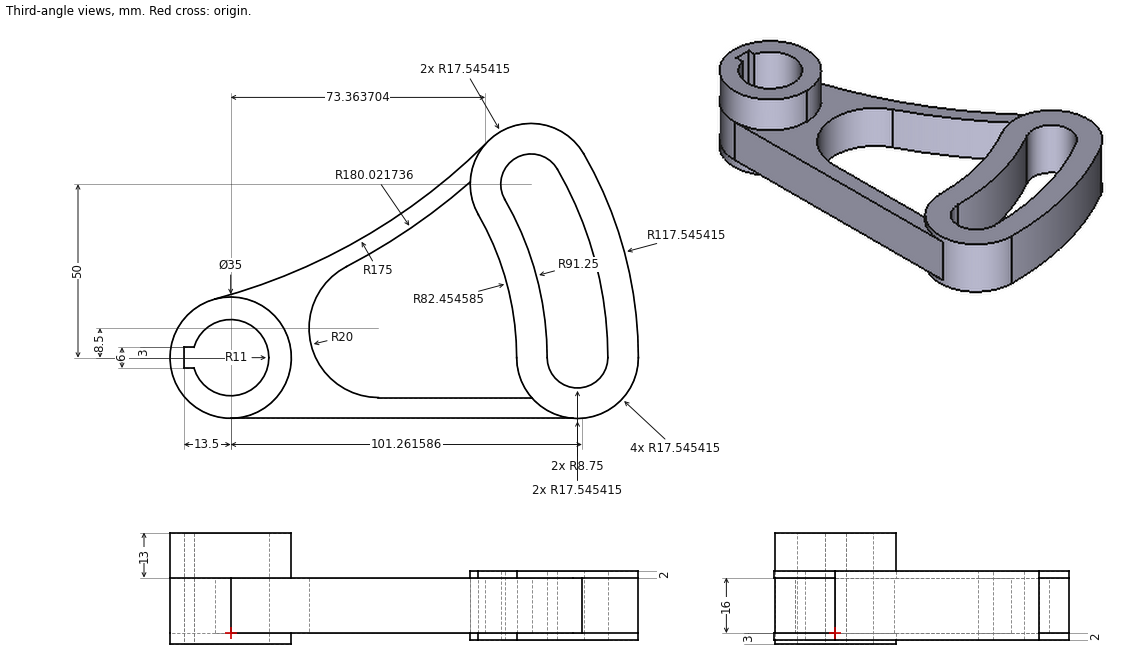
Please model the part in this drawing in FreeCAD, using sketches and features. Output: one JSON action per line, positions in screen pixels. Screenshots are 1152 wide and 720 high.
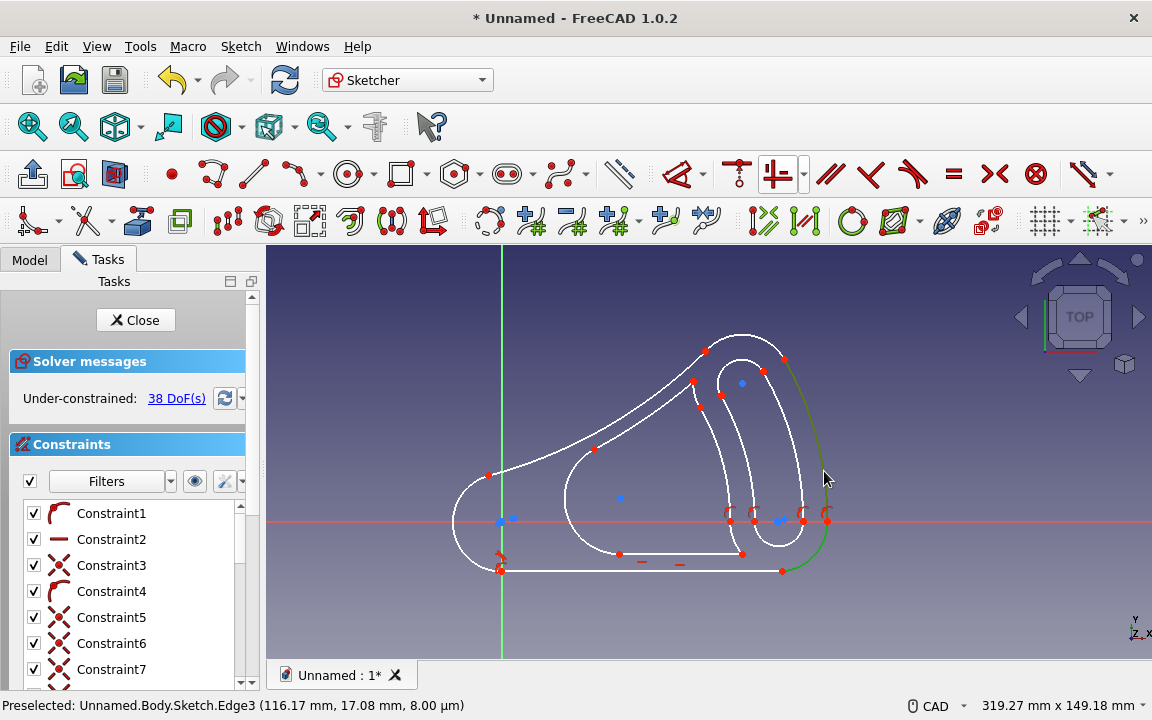
{"action": "left_click", "coordinate": [913, 174]}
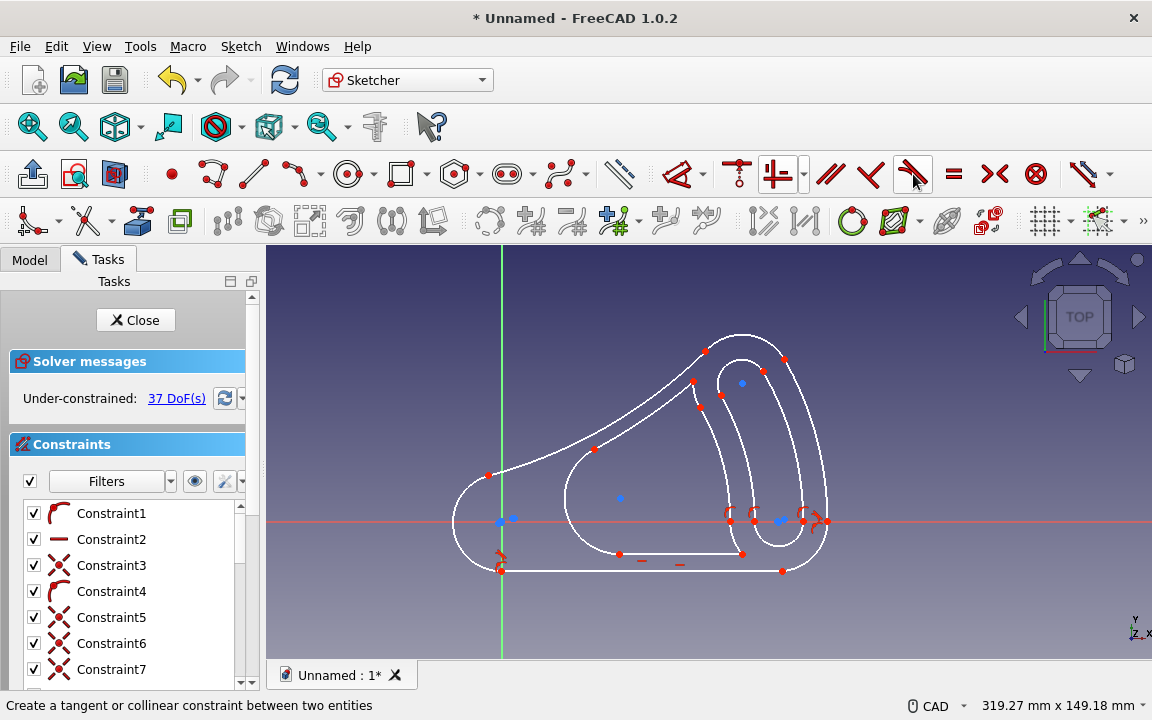
{"action": "left_click", "coordinate": [824, 471]}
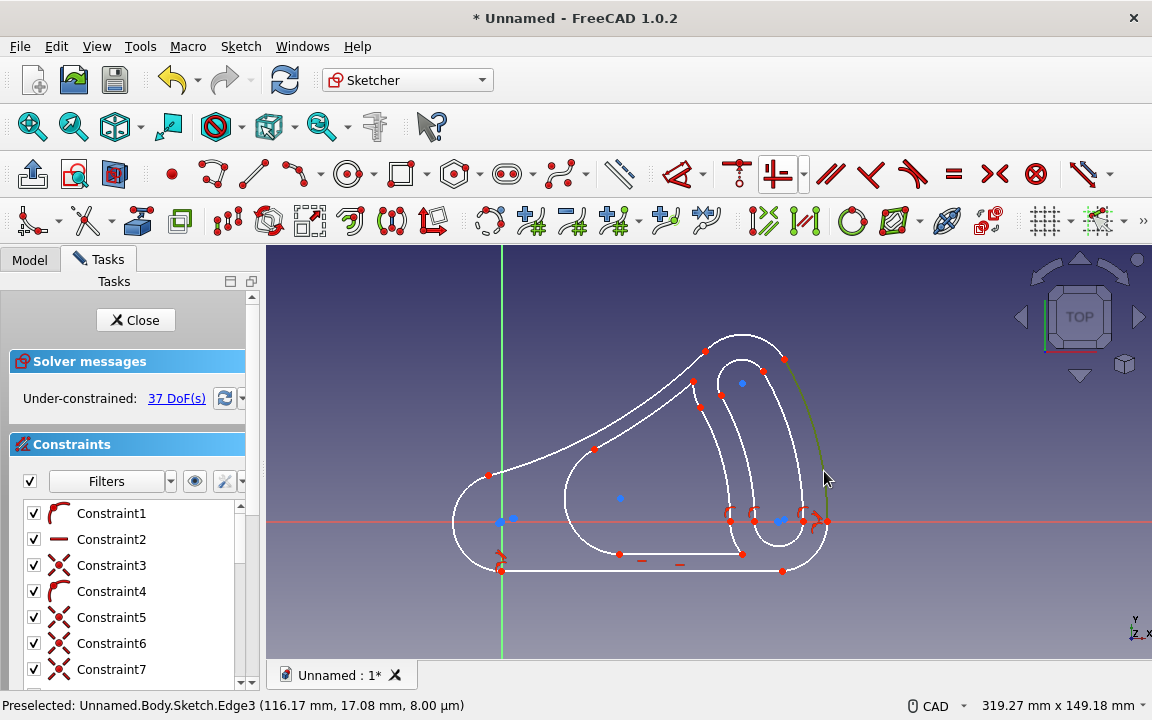
{"action": "left_click", "coordinate": [765, 340]}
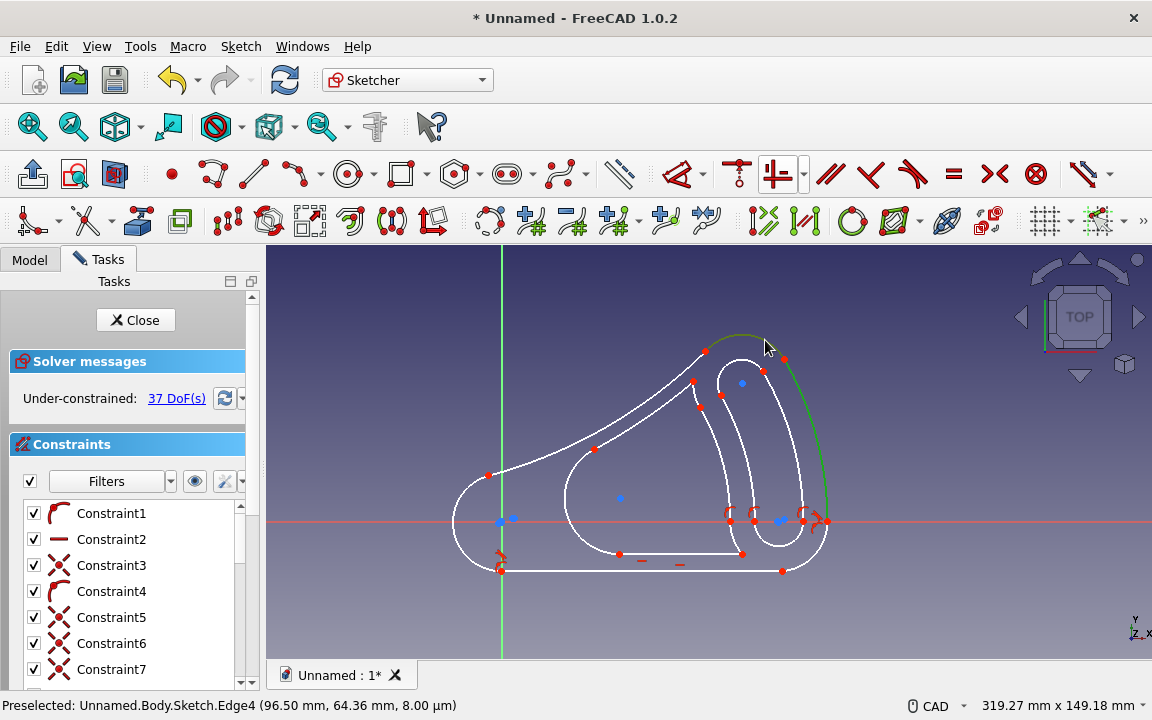
{"action": "left_click", "coordinate": [913, 174]}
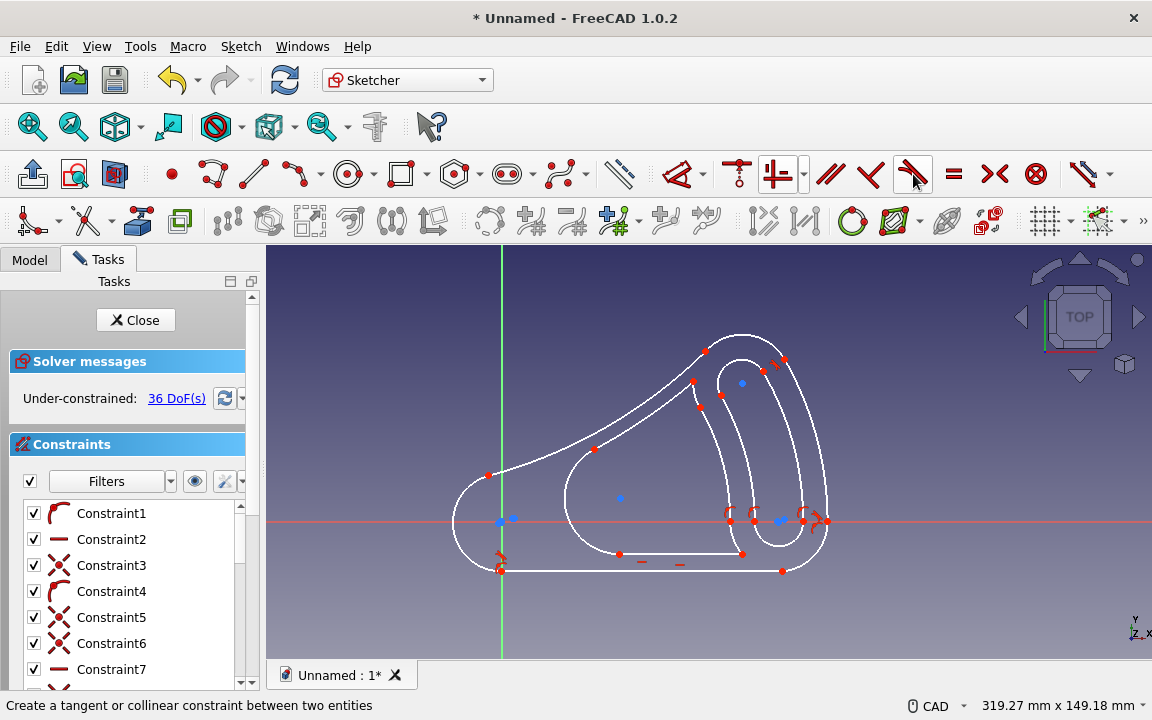
{"action": "left_click", "coordinate": [560, 451]}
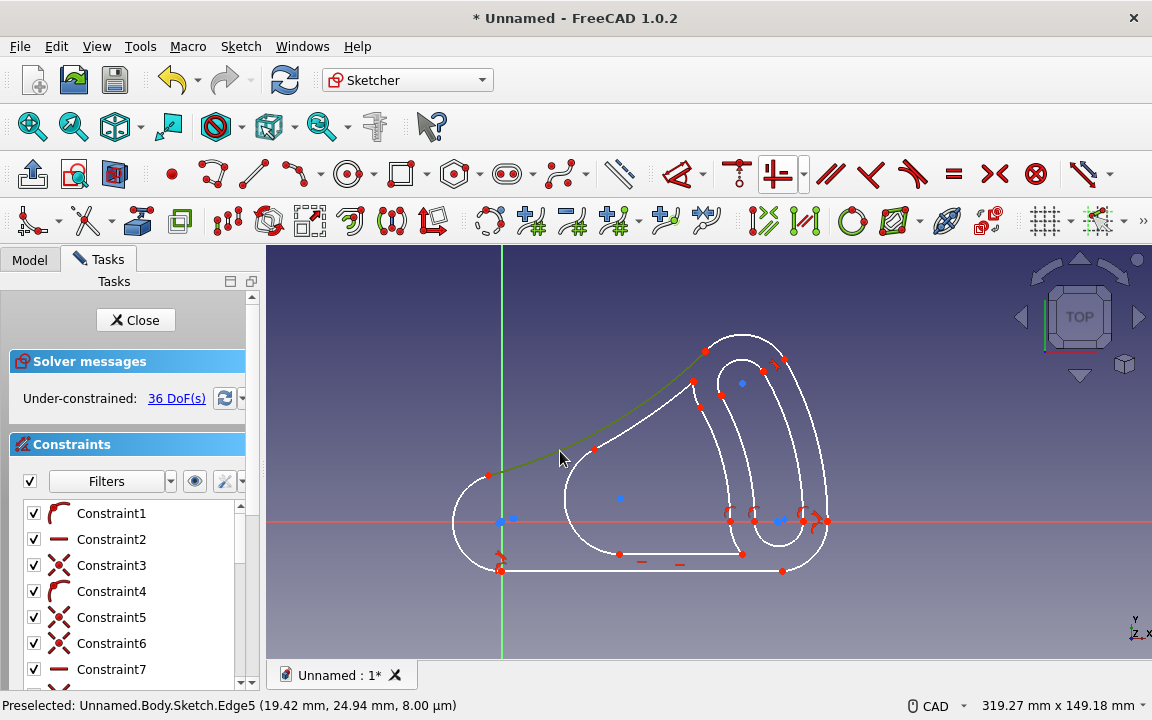
{"action": "left_click", "coordinate": [458, 502]}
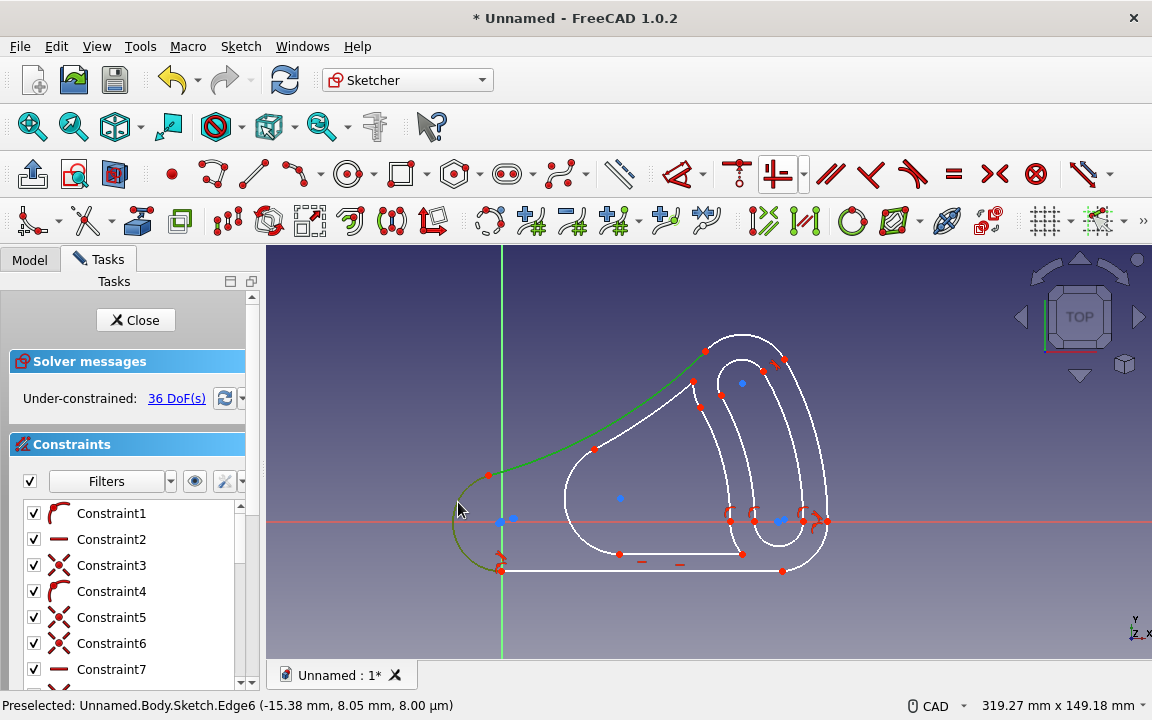
{"action": "left_click", "coordinate": [913, 174]}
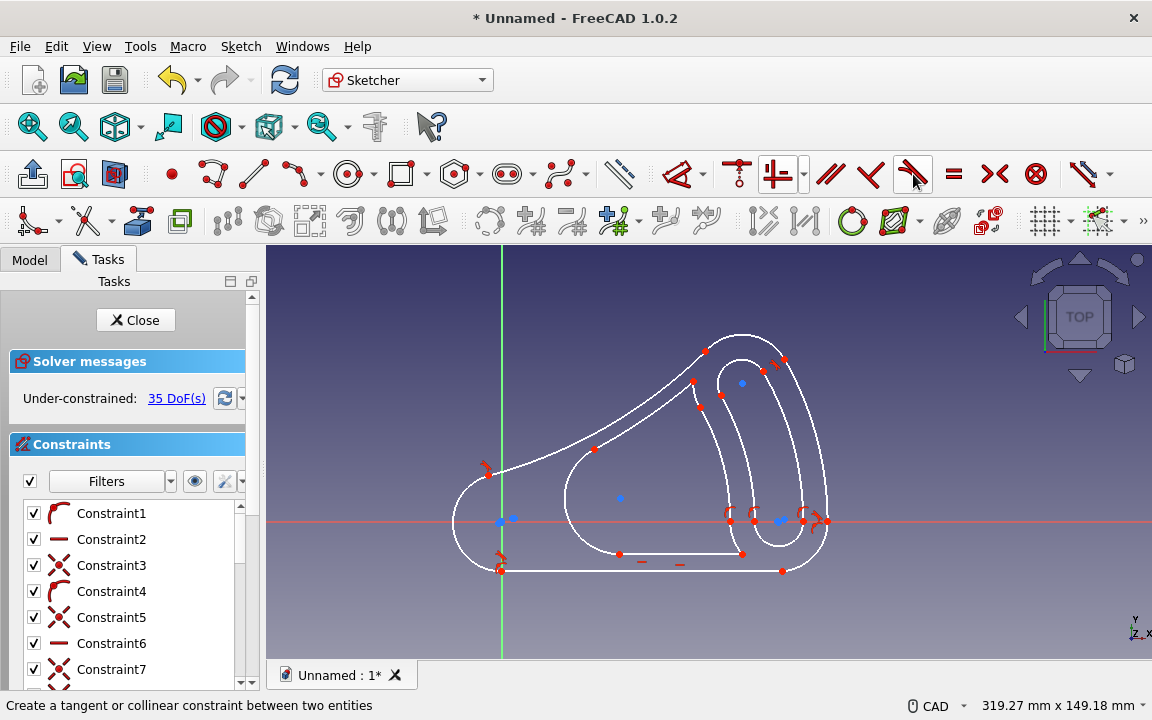
{"action": "left_click", "coordinate": [705, 554]}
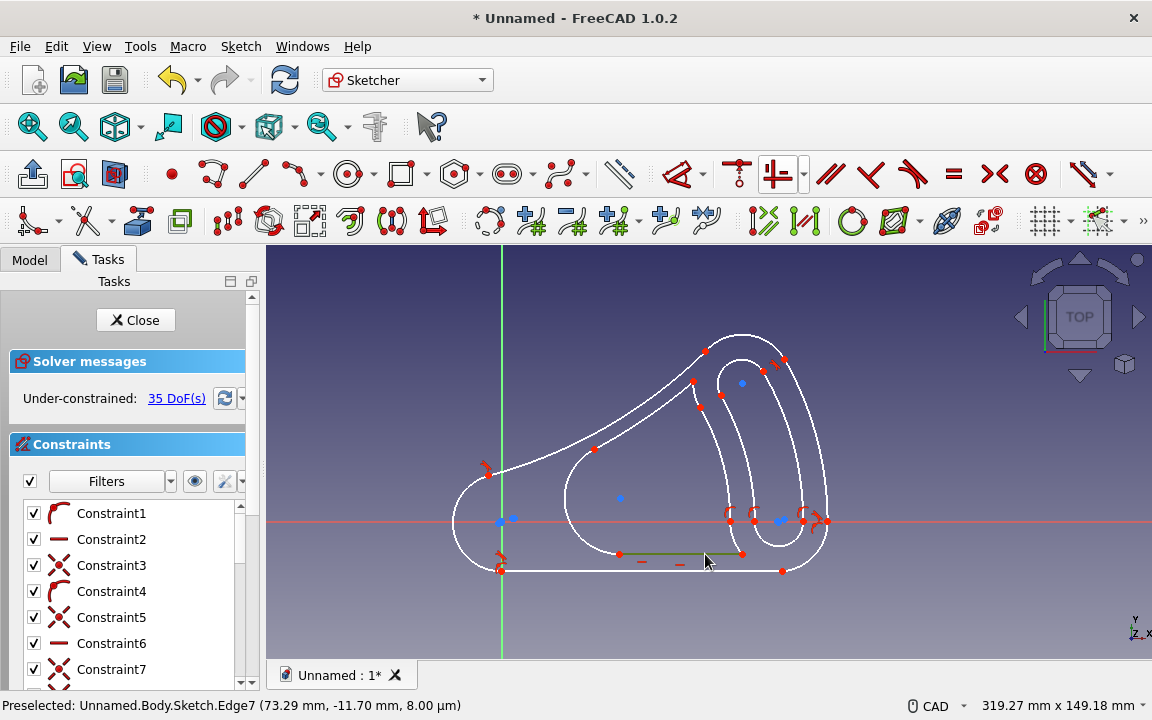
{"action": "left_click", "coordinate": [567, 483]}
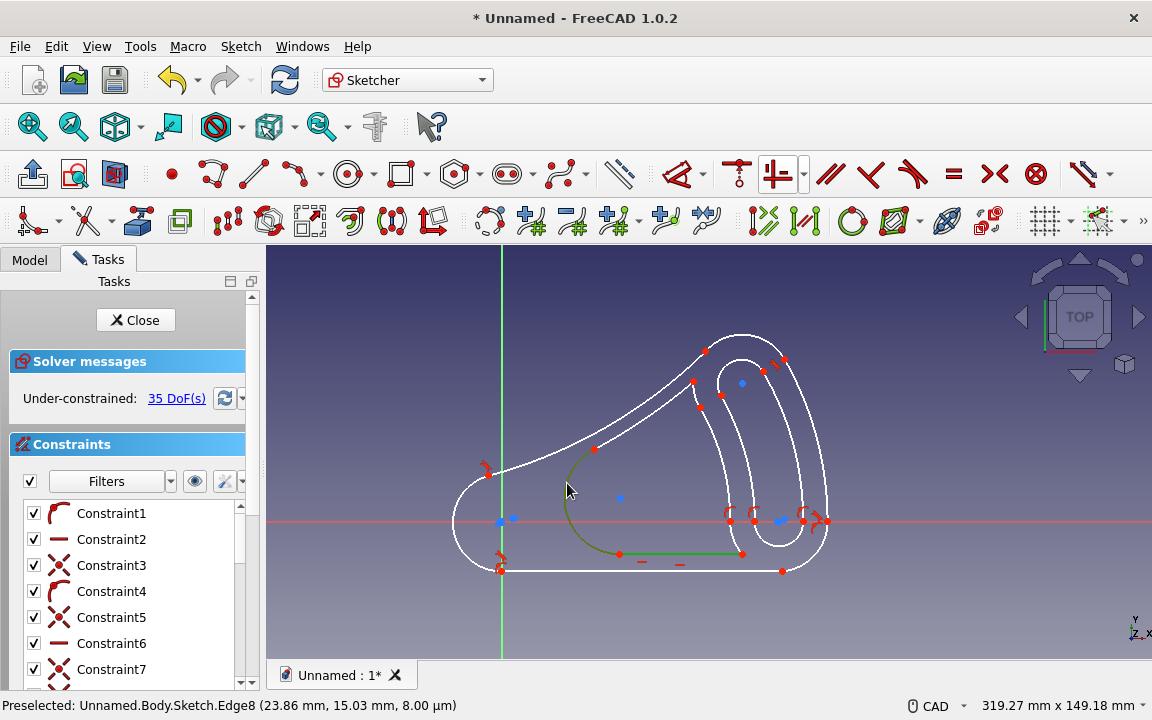
{"action": "left_click", "coordinate": [913, 174]}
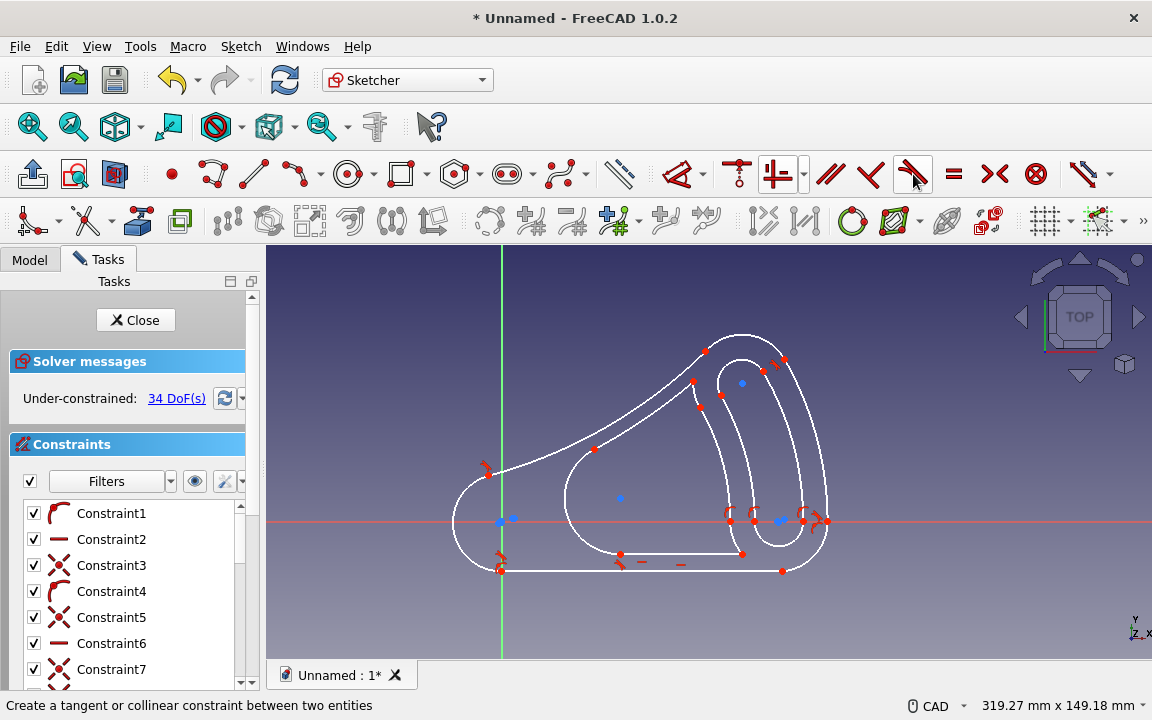
{"action": "left_click", "coordinate": [567, 483]}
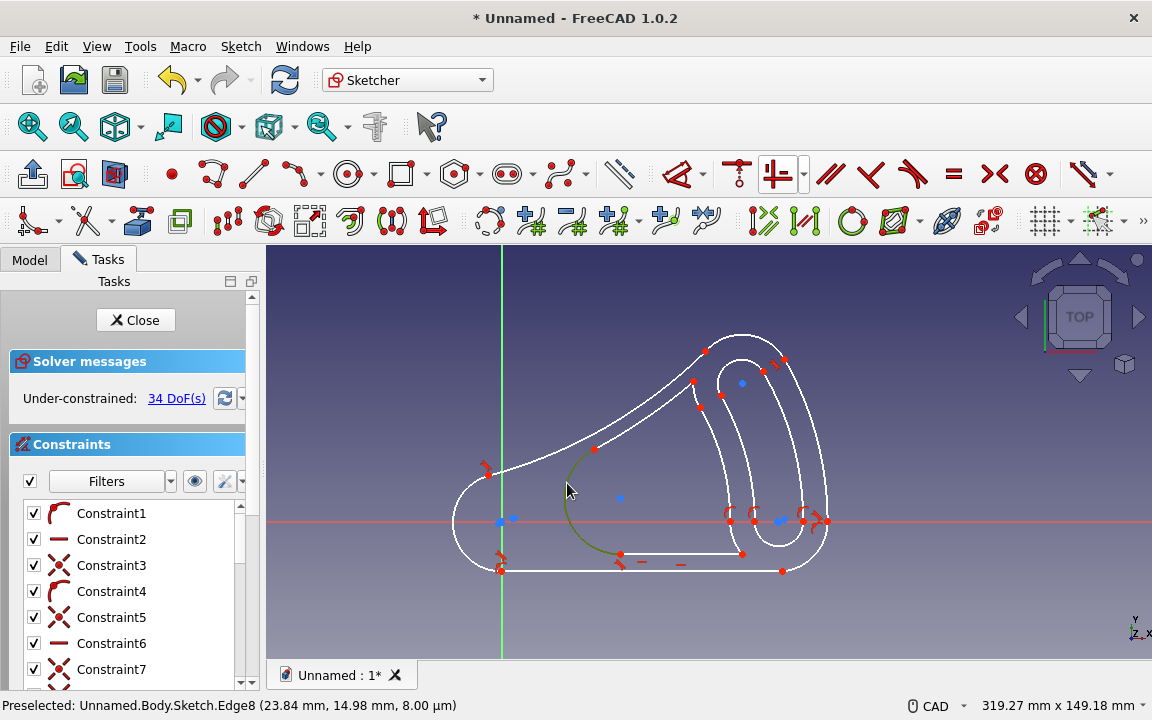
{"action": "left_click", "coordinate": [625, 432]}